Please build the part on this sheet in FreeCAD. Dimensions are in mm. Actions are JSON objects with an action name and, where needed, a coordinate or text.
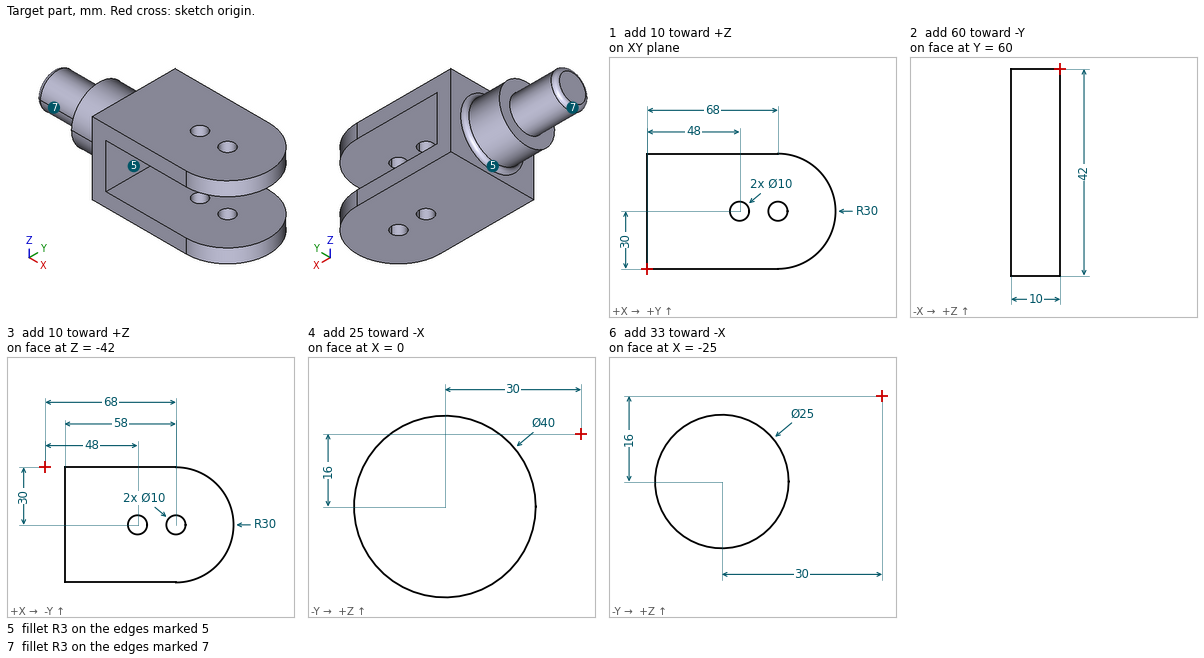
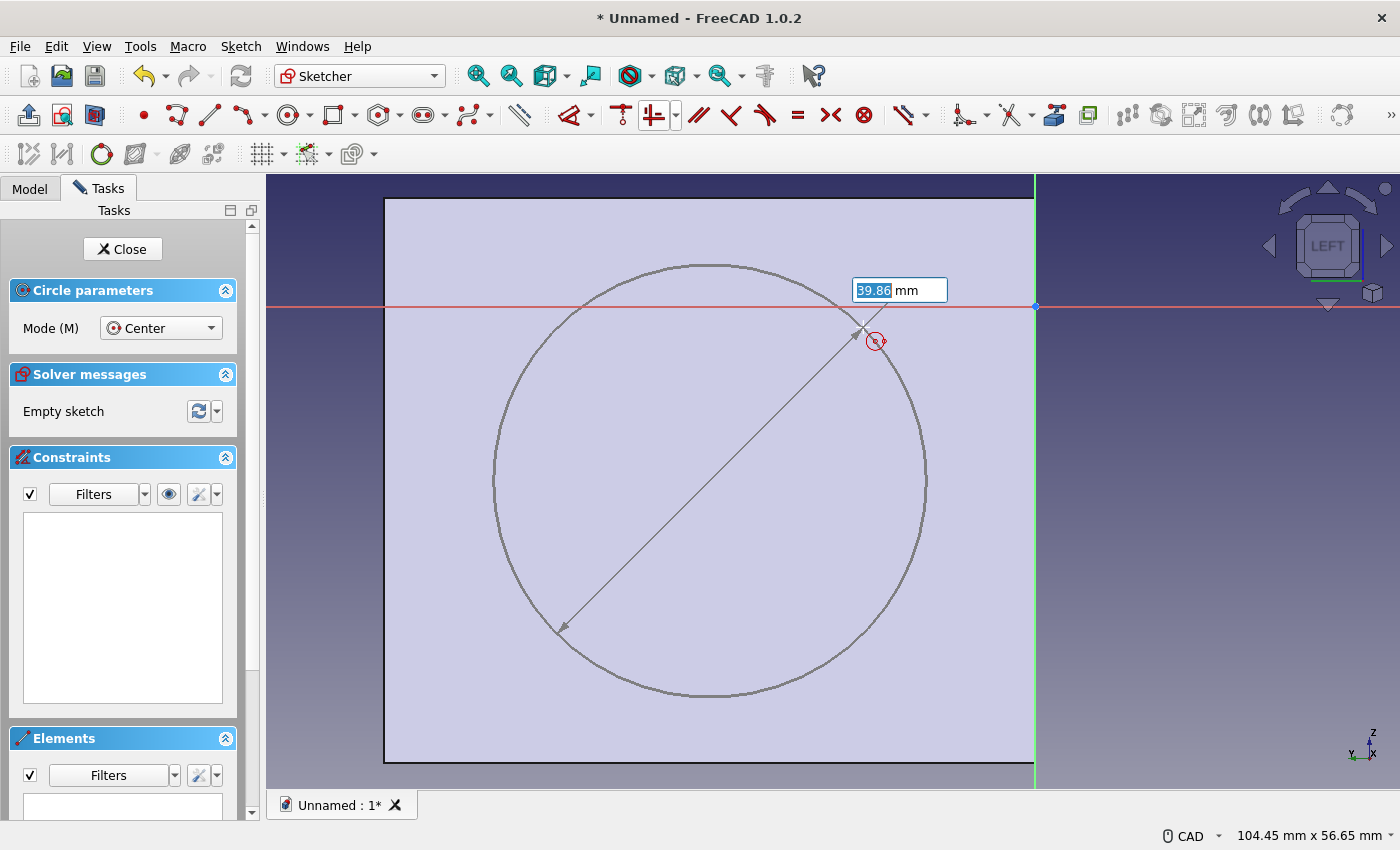
{"action": "type", "text": "40"}
{"action": "key", "text": "Return"}
{"action": "key", "text": "Escape"}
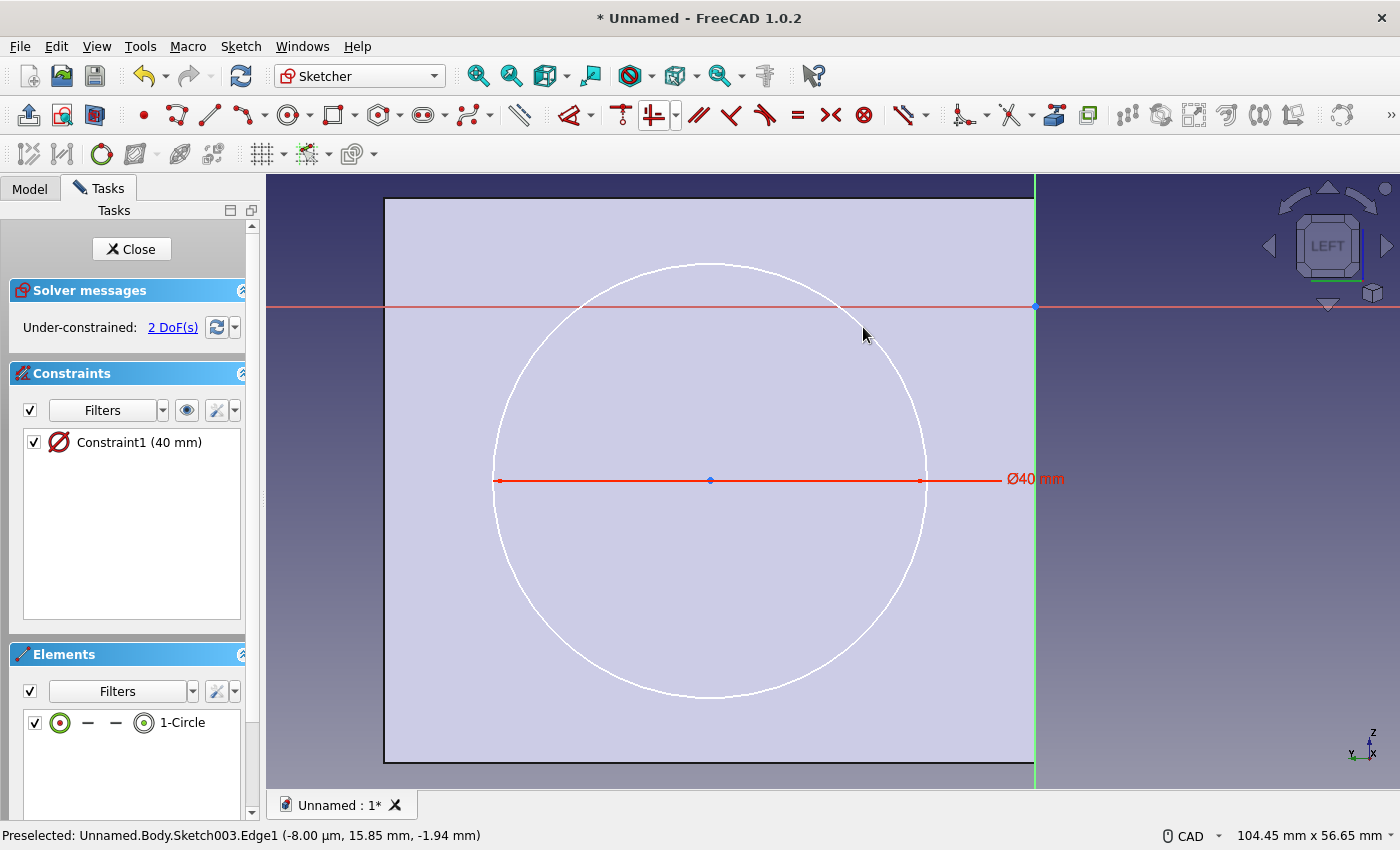
{"action": "key", "text": "d"}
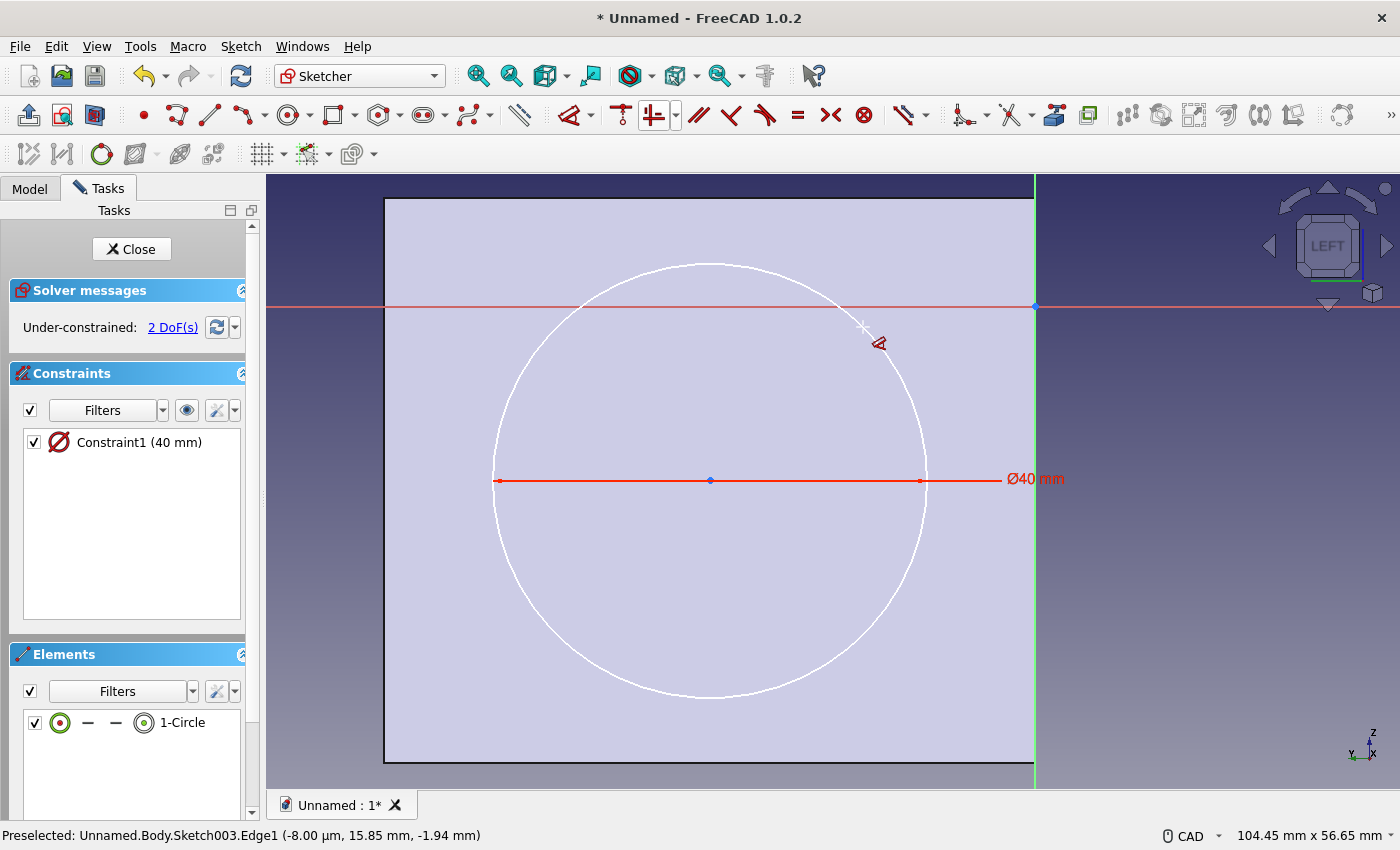
{"action": "left_click", "coordinate": [710, 481]}
{"action": "left_click", "coordinate": [873, 273]}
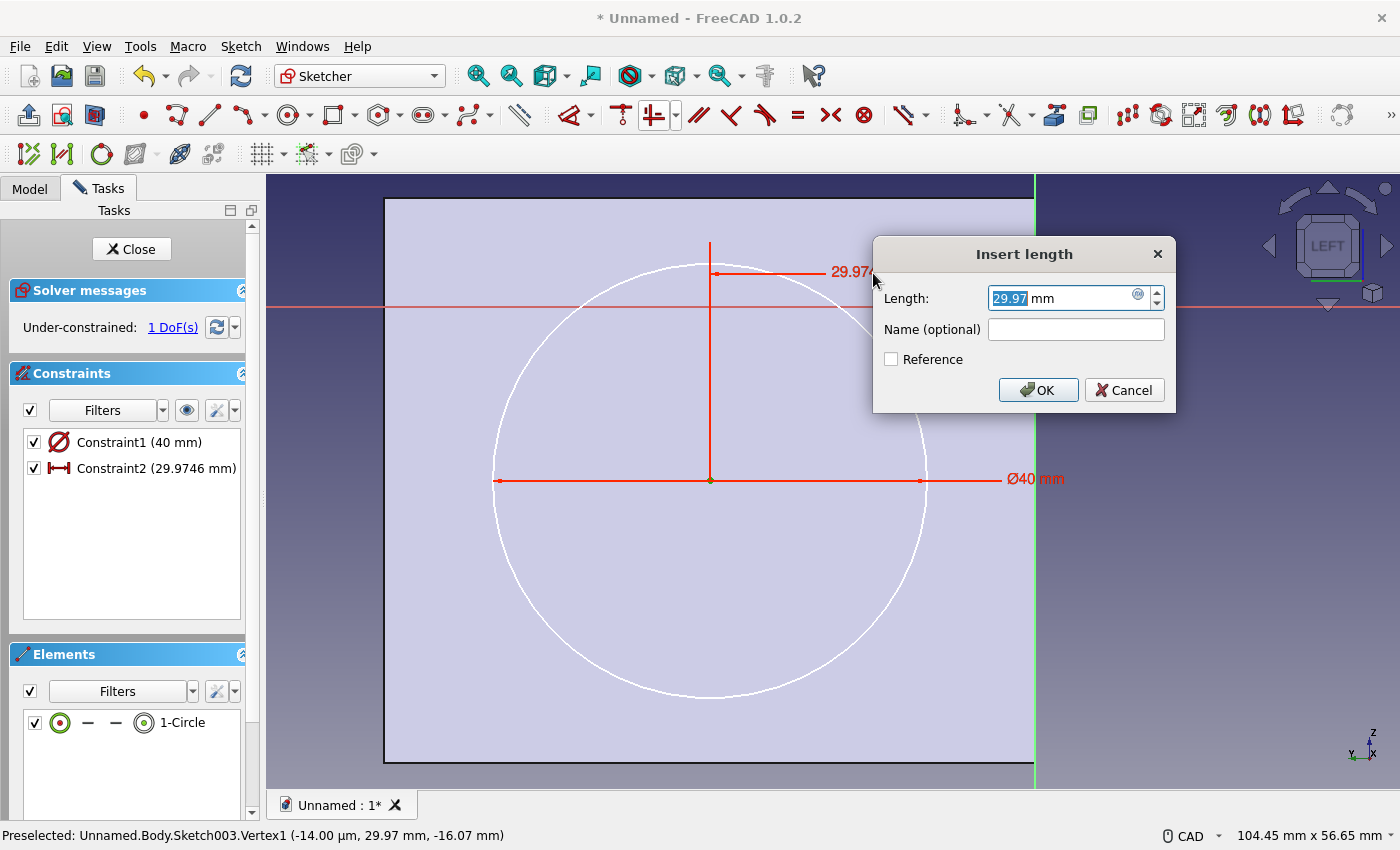
{"action": "type", "text": "30"}
{"action": "key", "text": "Return"}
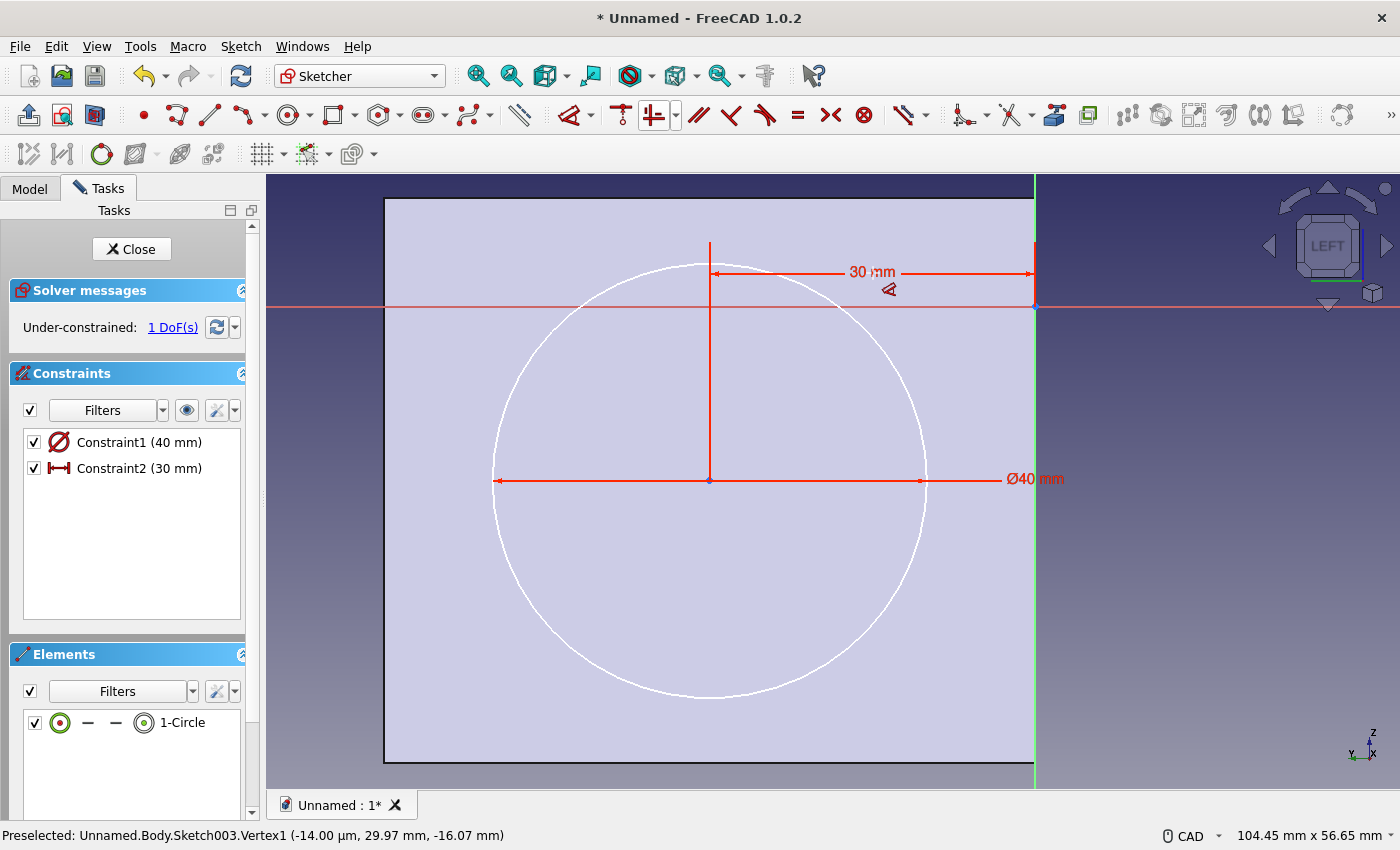
{"action": "left_click", "coordinate": [710, 481]}
{"action": "left_click", "coordinate": [1069, 394]}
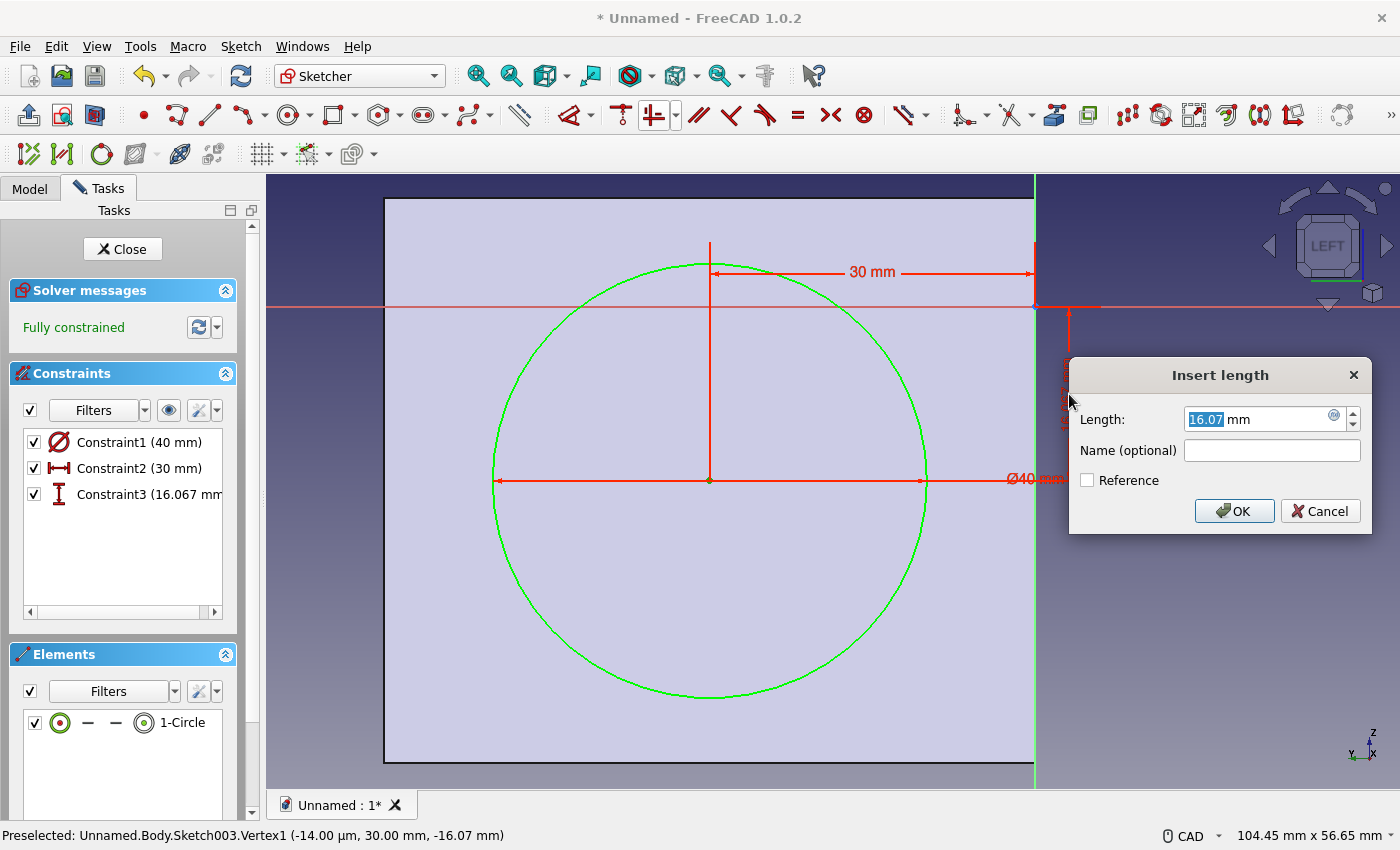
{"action": "type", "text": "16"}
{"action": "key", "text": "Return"}
{"action": "key", "text": "Escape"}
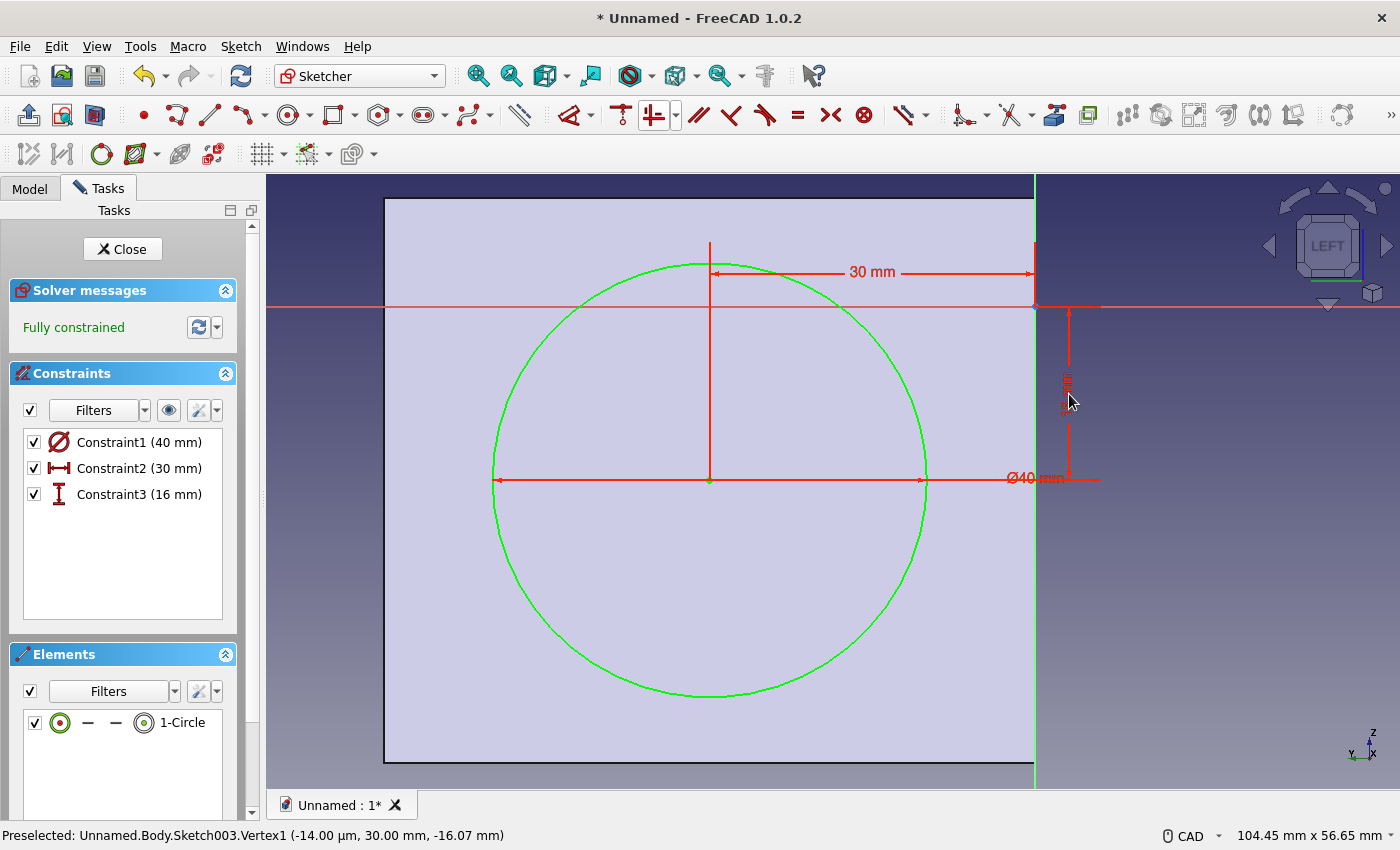
{"action": "left_click", "coordinate": [123, 249]}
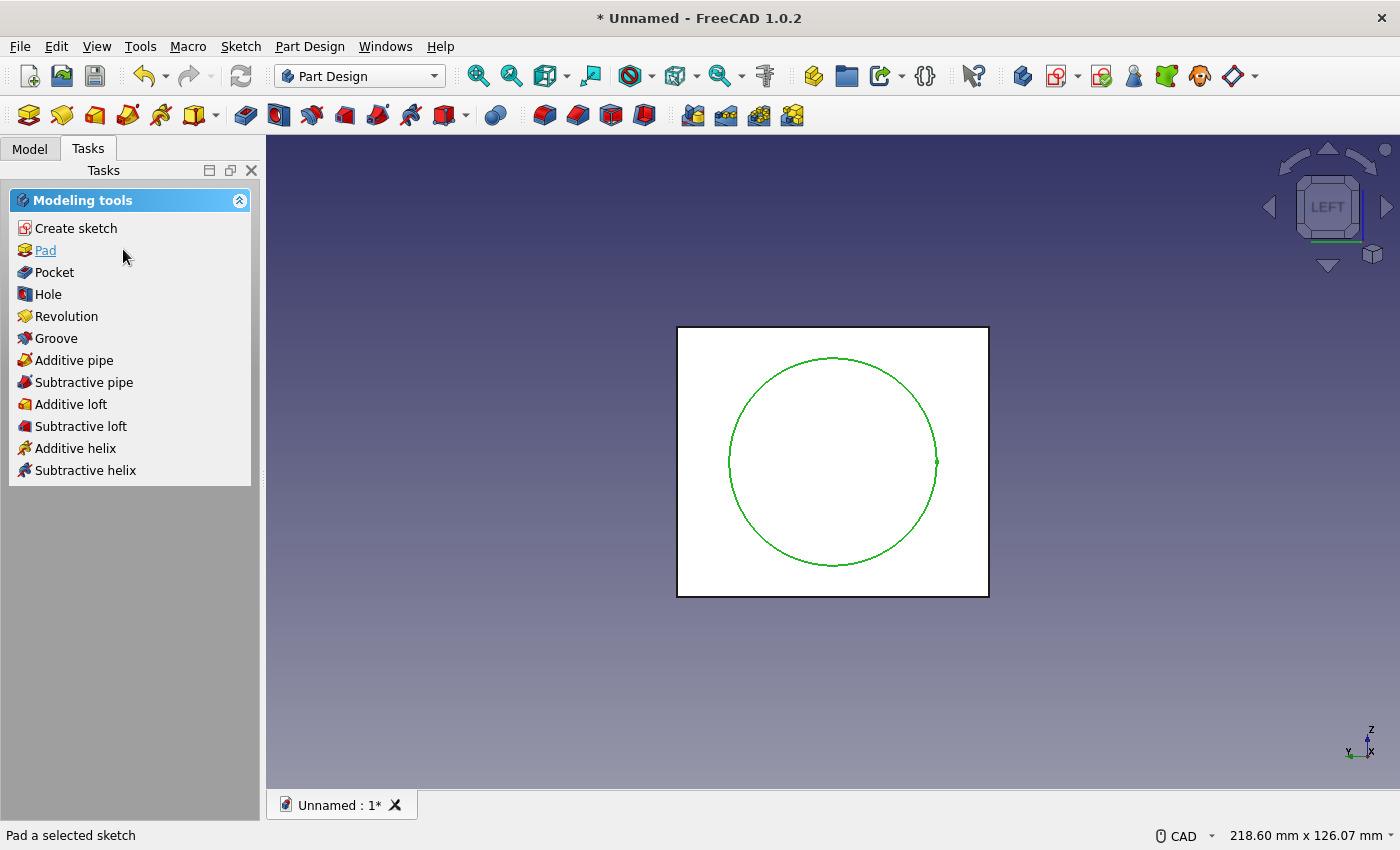
{"action": "left_click", "coordinate": [29, 116]}